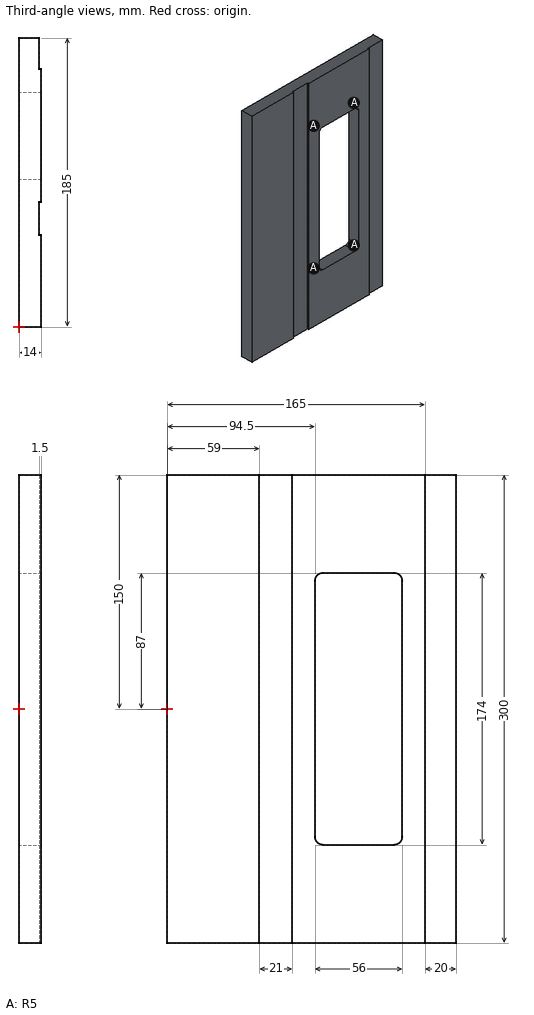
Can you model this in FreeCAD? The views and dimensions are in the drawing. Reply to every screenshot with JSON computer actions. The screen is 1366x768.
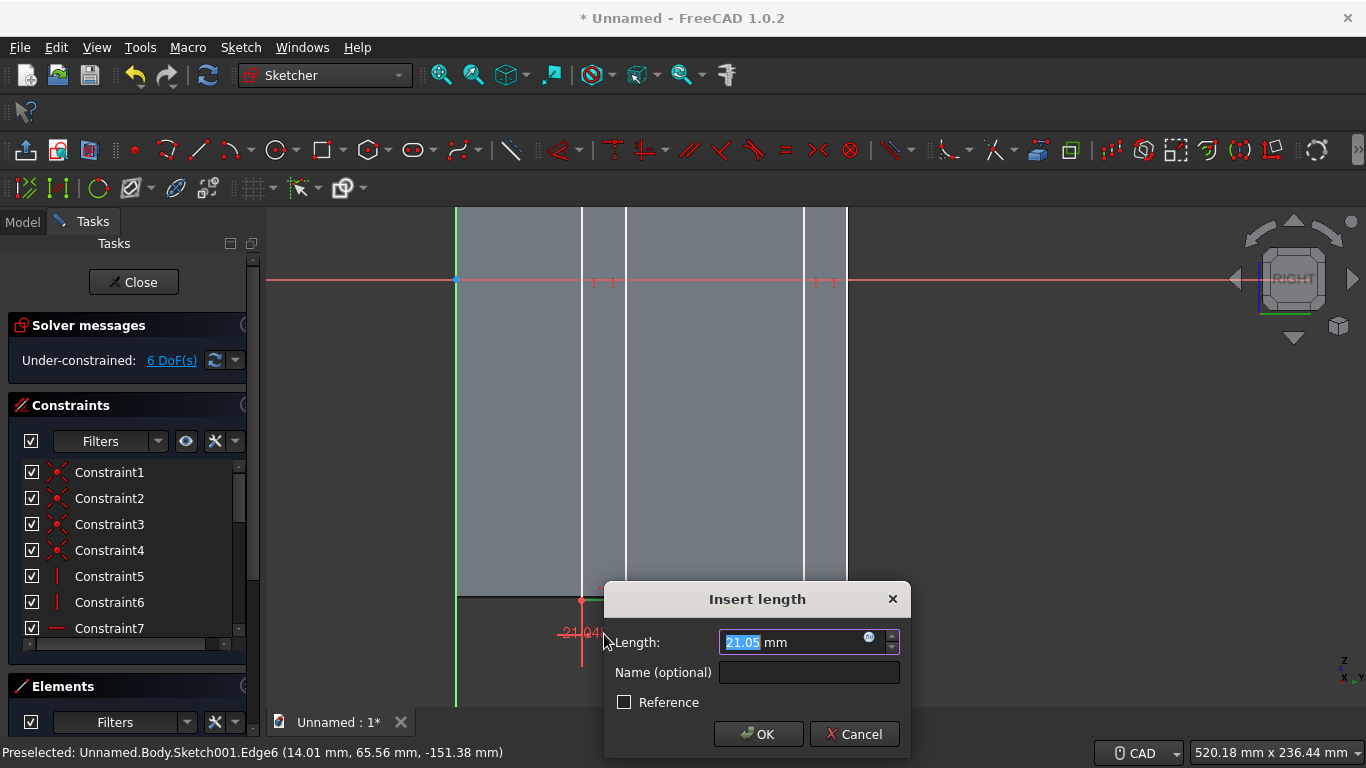
{"action": "type", "text": "21"}
{"action": "key", "text": "Return"}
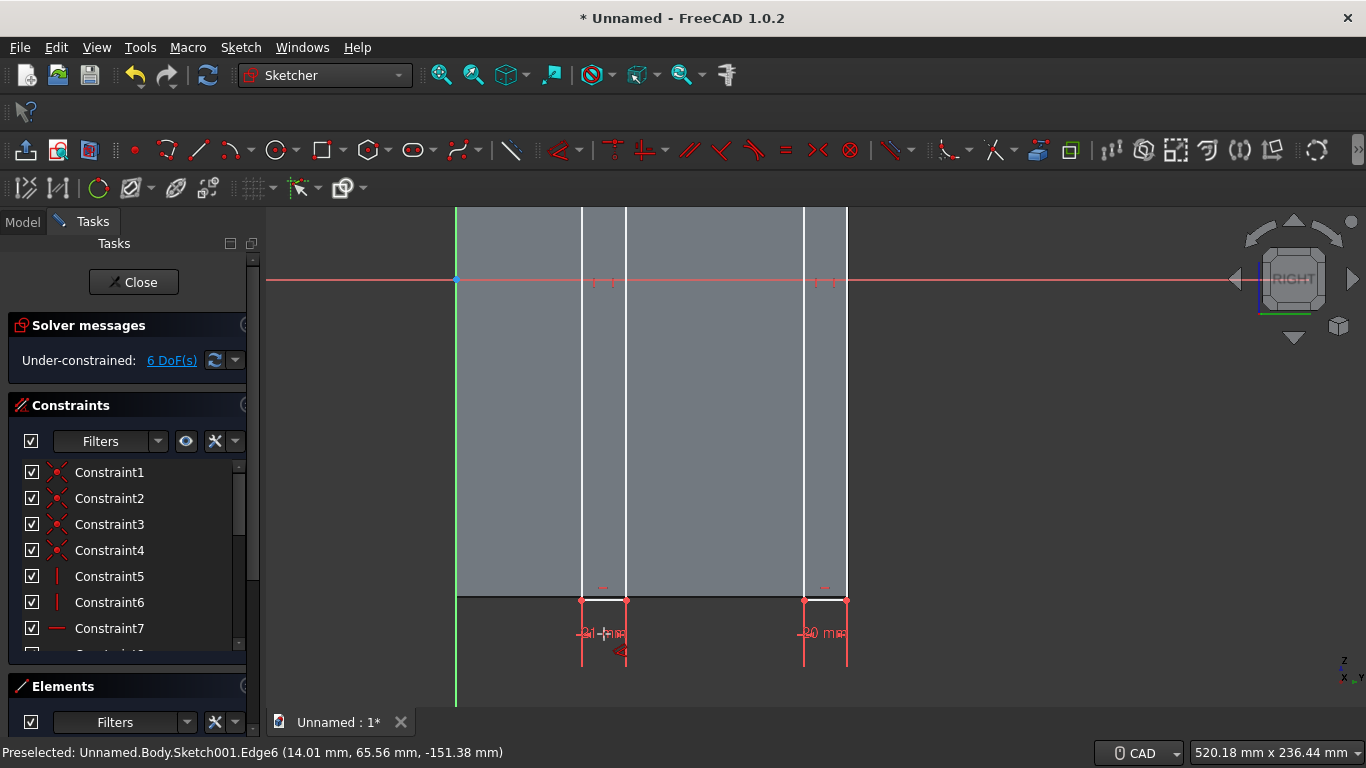
{"action": "left_click", "coordinate": [804, 410]}
{"action": "left_click", "coordinate": [770, 418]}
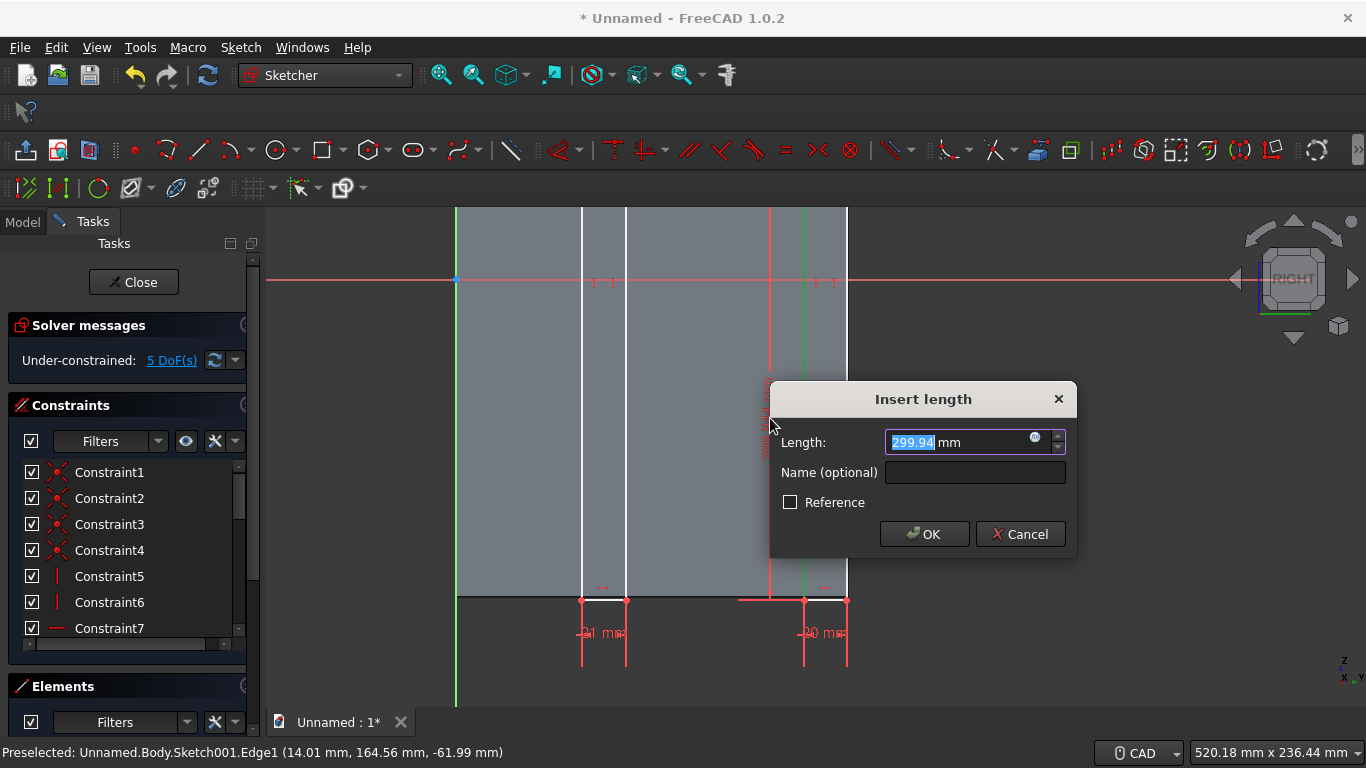
{"action": "type", "text": "300"}
{"action": "key", "text": "Return"}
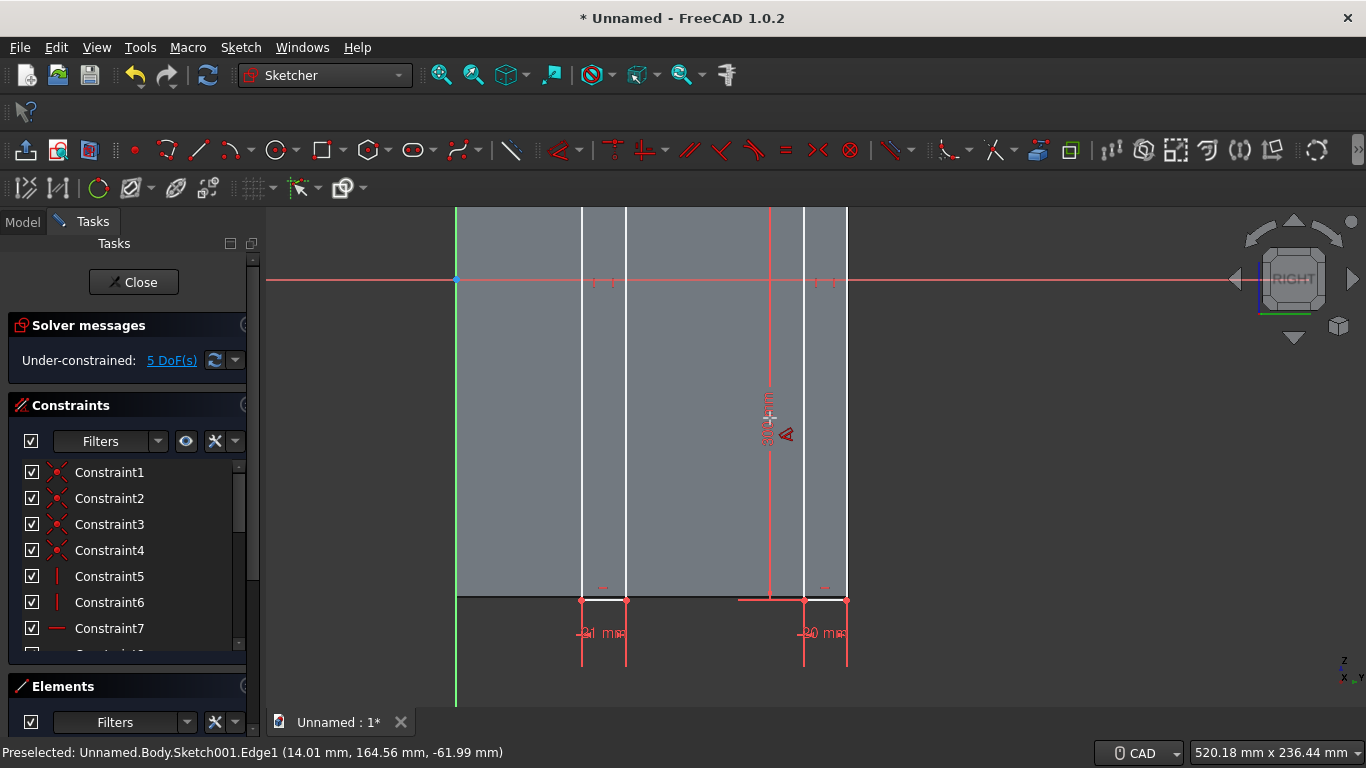
{"action": "left_click", "coordinate": [582, 410]}
{"action": "left_click", "coordinate": [548, 418]}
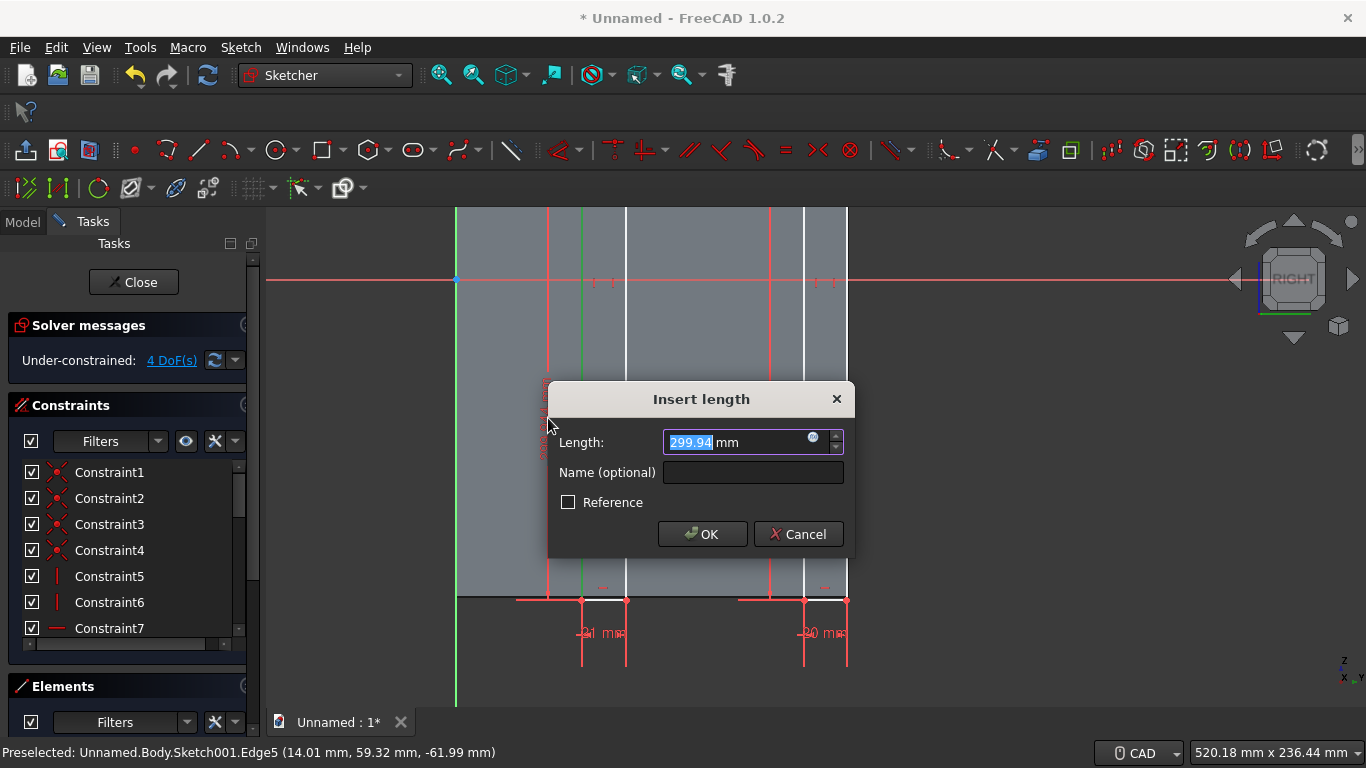
{"action": "type", "text": "300"}
{"action": "key", "text": "Return"}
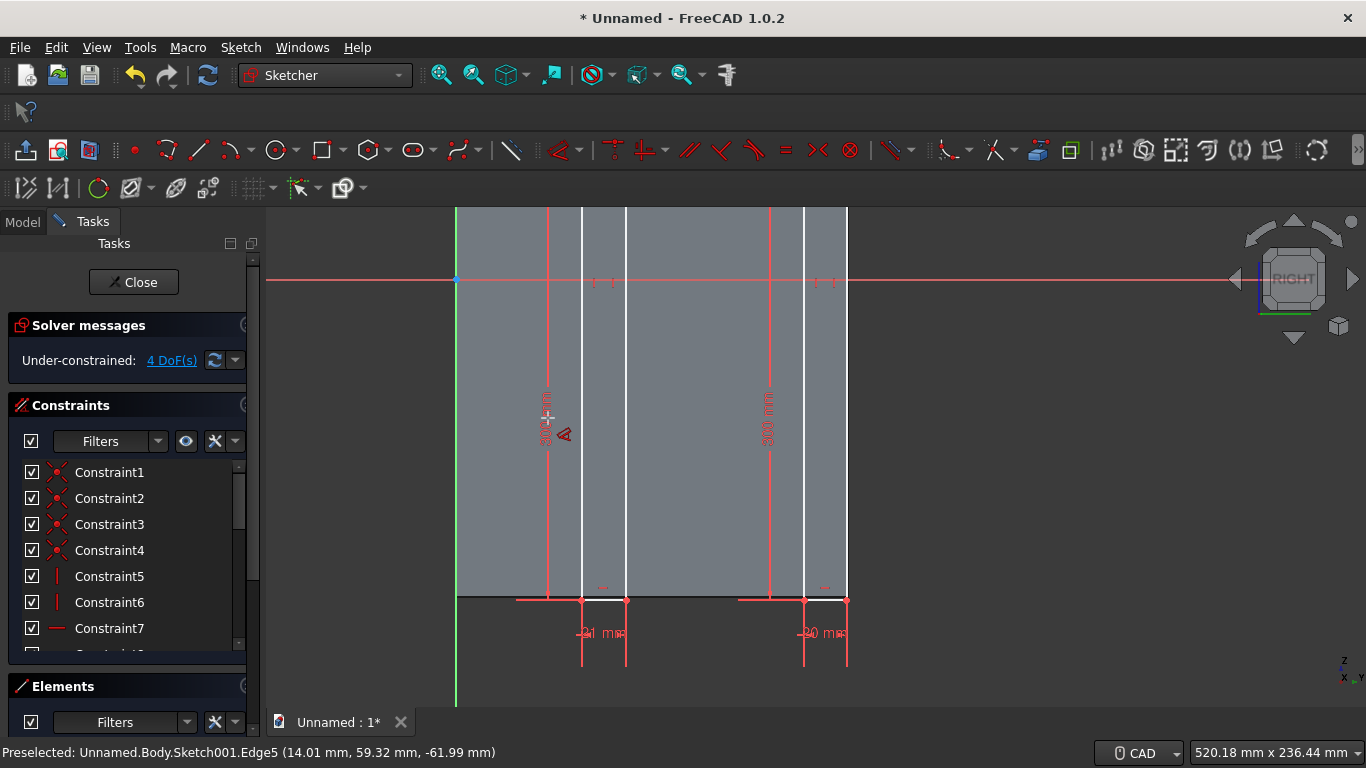
{"action": "scroll", "coordinate": [825, 601], "scroll_direction": "down", "scroll_amount": 4}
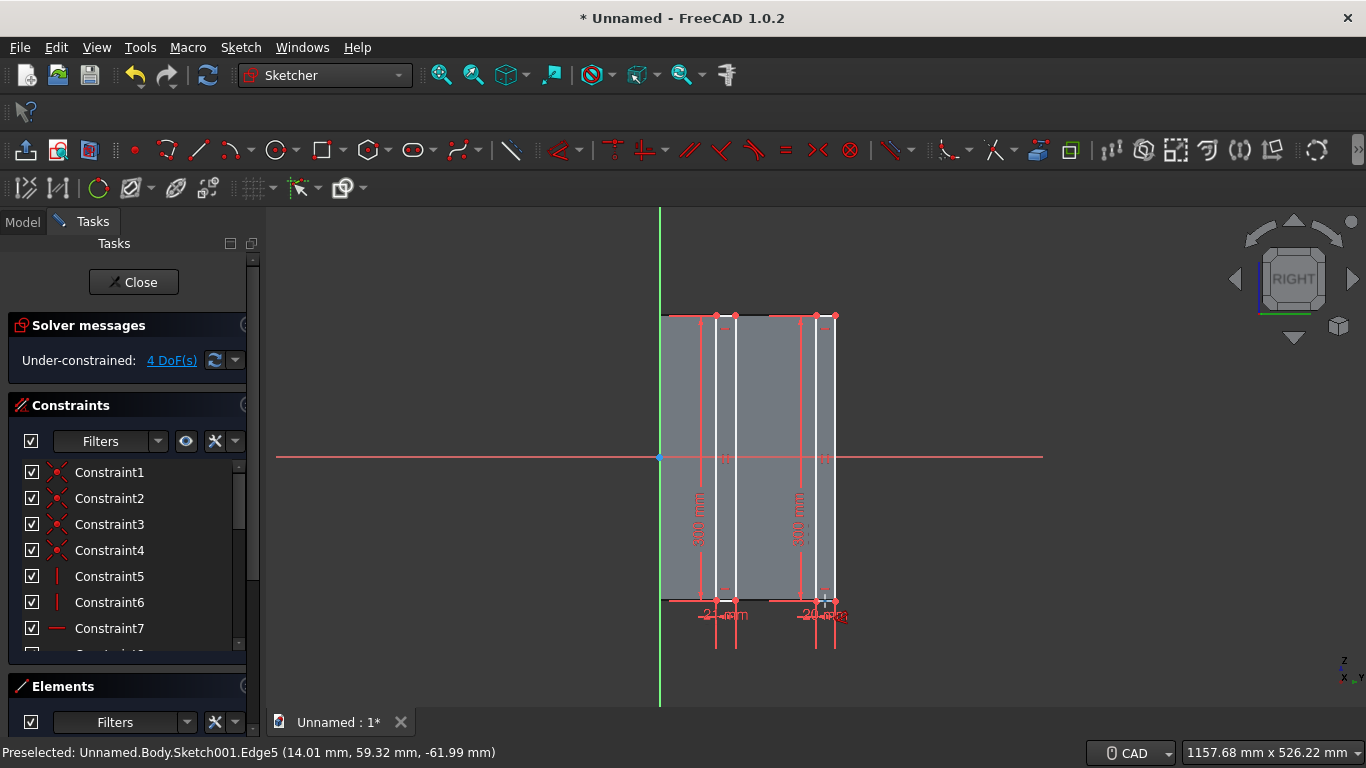
{"action": "left_click", "coordinate": [716, 316]}
{"action": "left_click", "coordinate": [688, 282]}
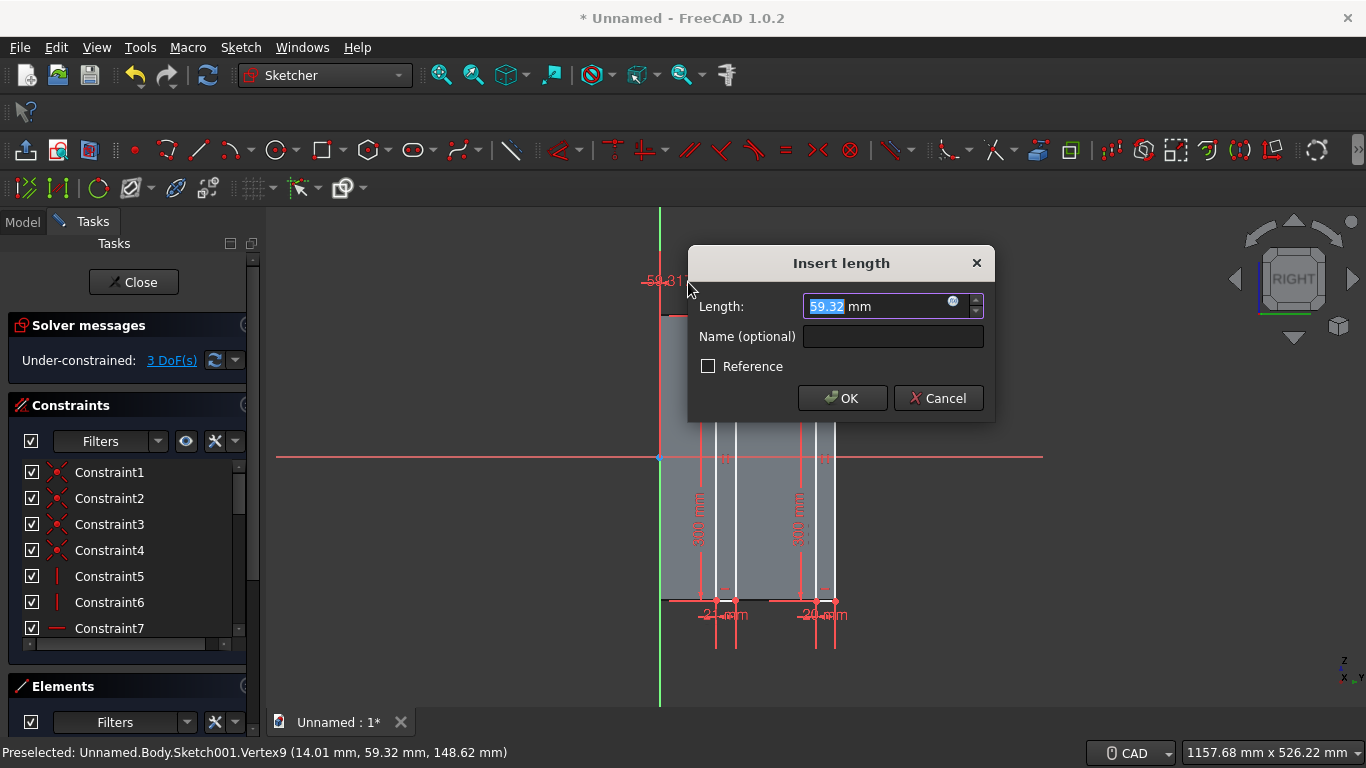
{"action": "type", "text": "59"}
{"action": "key", "text": "Return"}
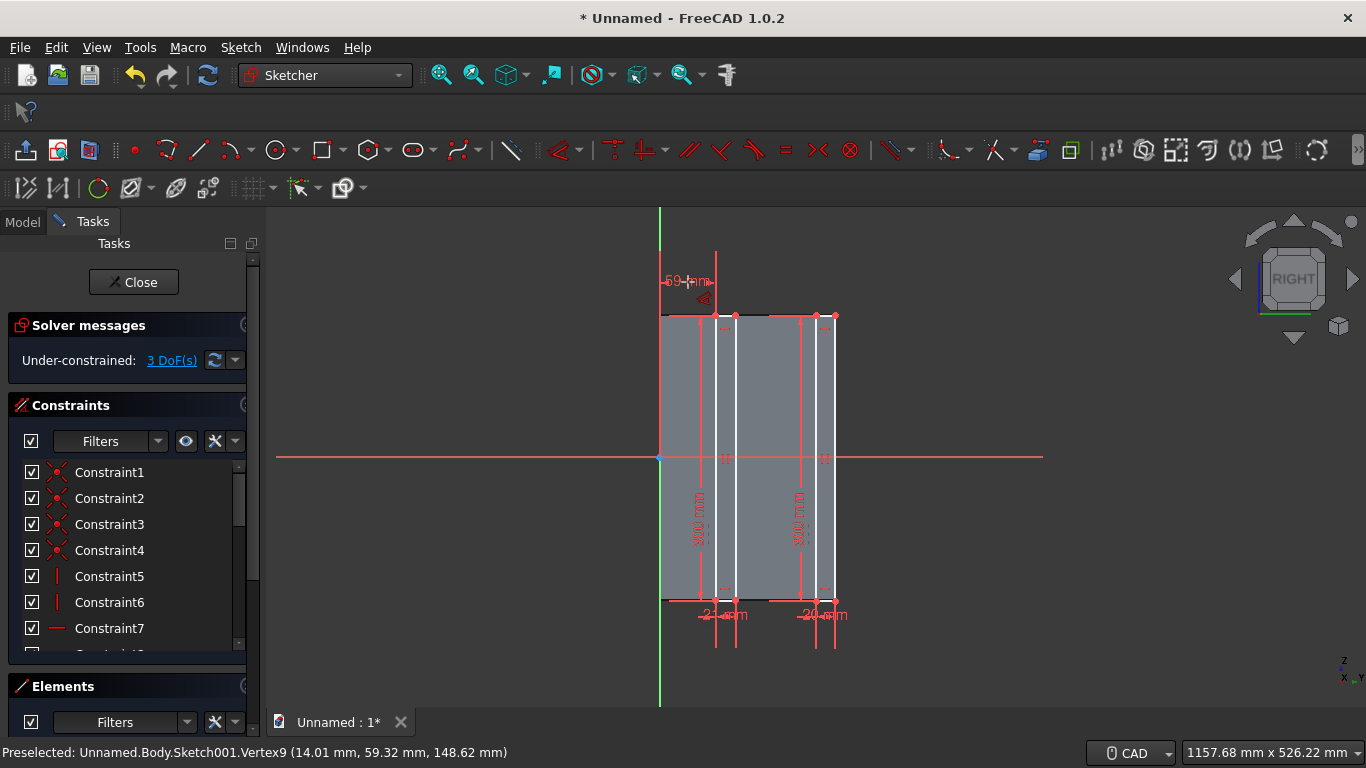
{"action": "left_click", "coordinate": [816, 316]}
{"action": "left_click", "coordinate": [774, 282]}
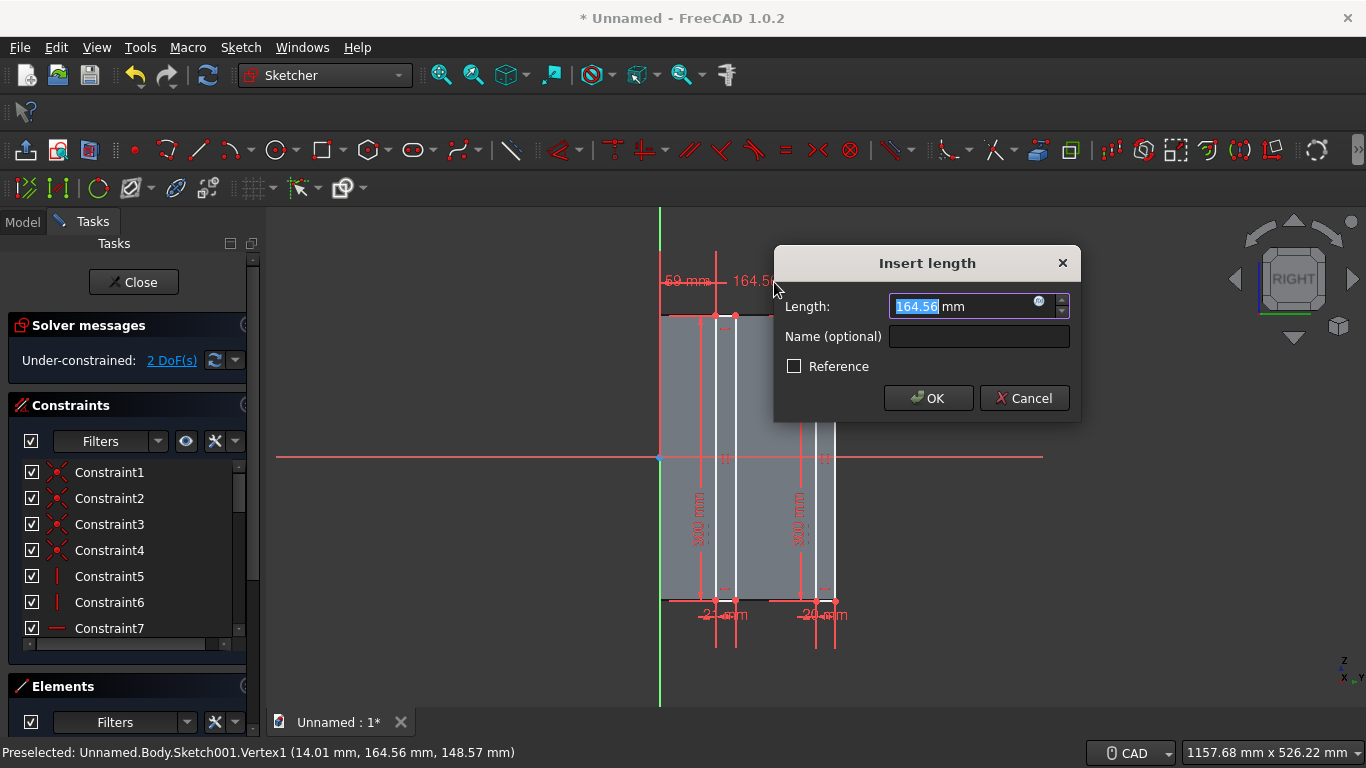
{"action": "type", "text": "165"}
{"action": "key", "text": "Return"}